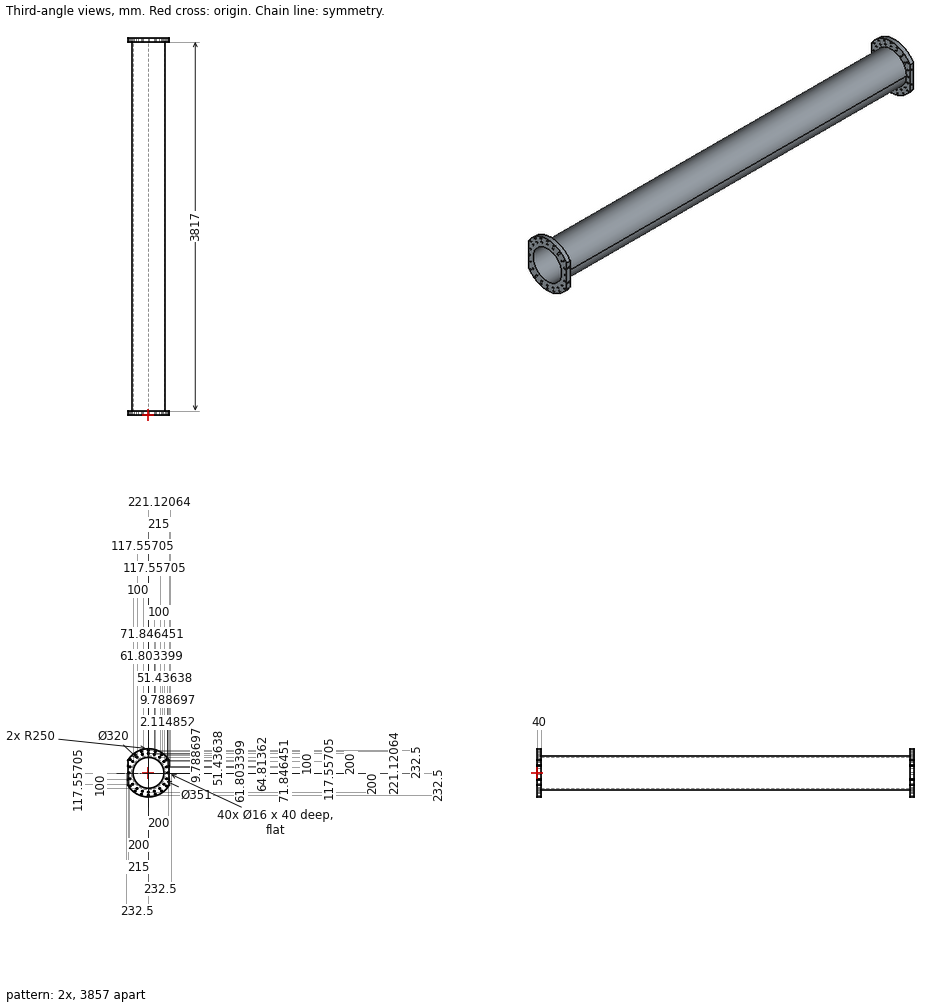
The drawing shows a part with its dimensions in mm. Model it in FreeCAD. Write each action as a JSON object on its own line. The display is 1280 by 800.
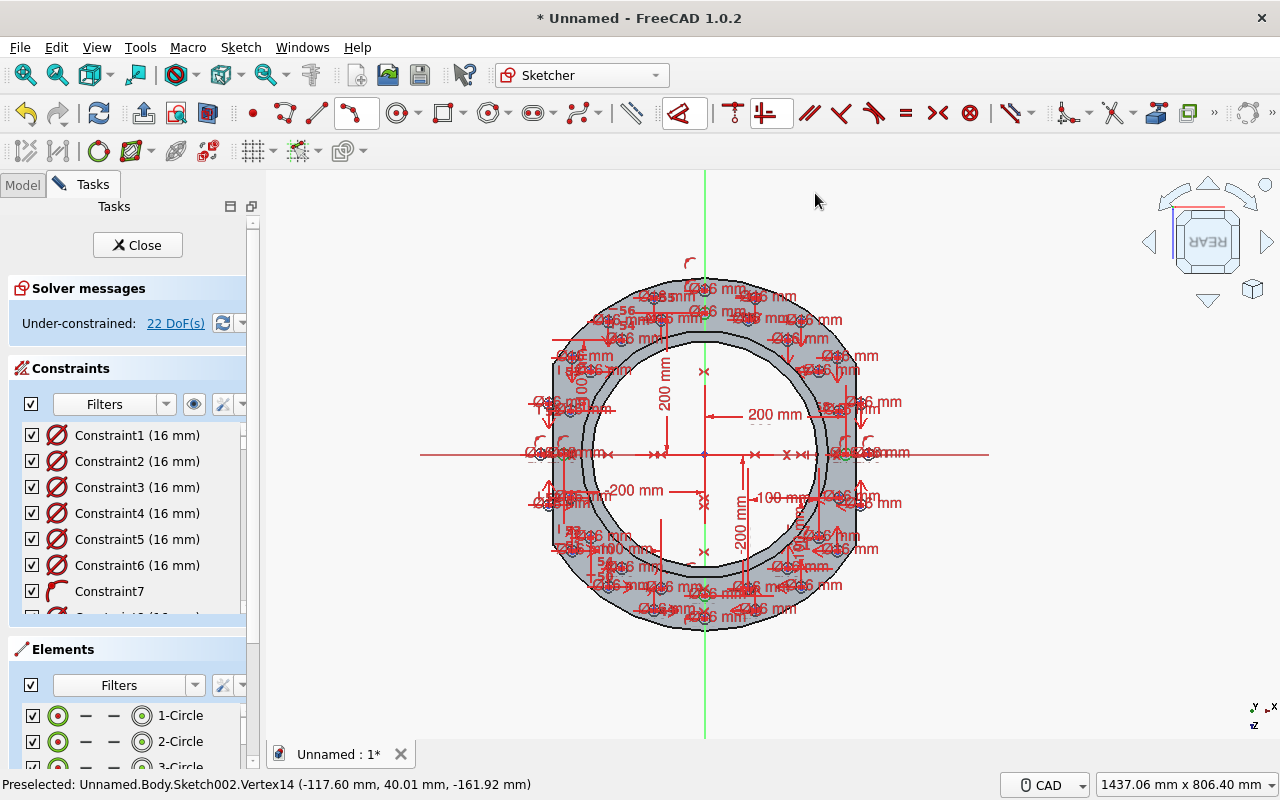
{"action": "scroll", "coordinate": [748, 320], "scroll_direction": "up", "scroll_amount": 4}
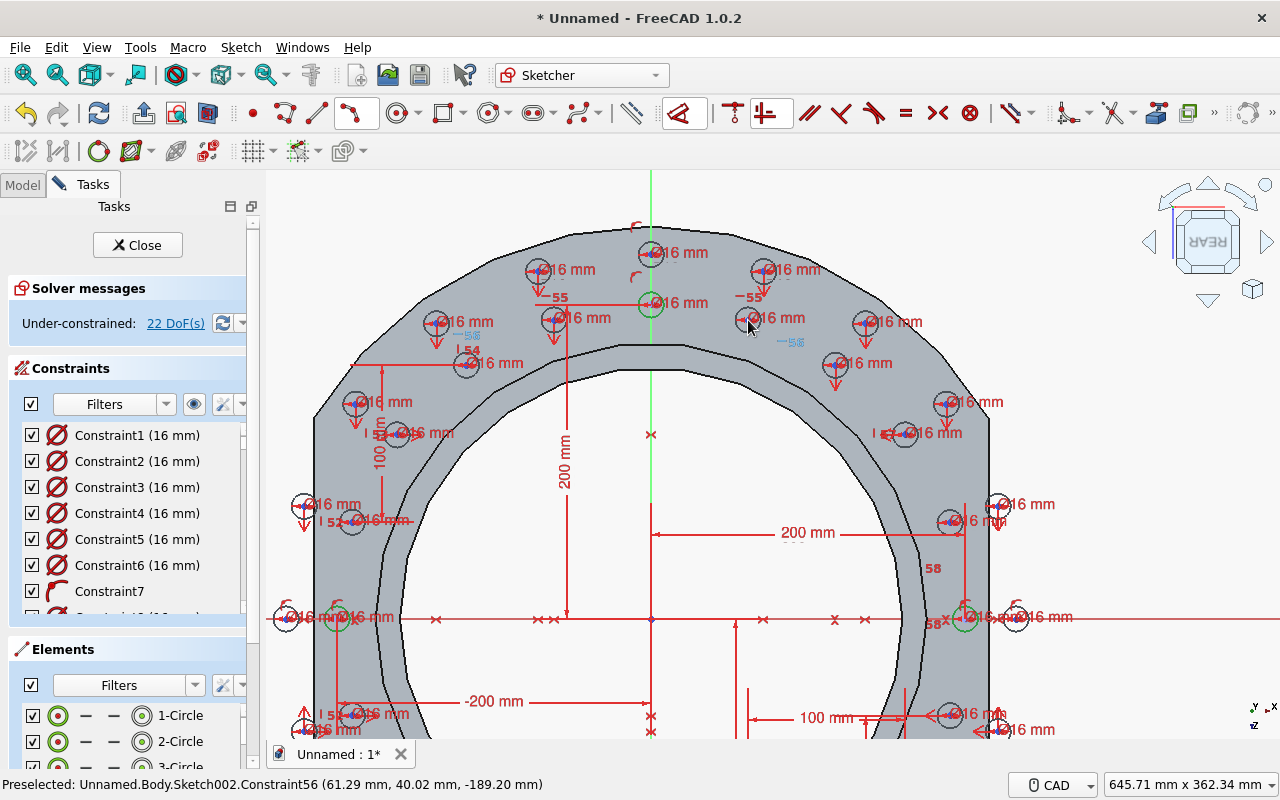
{"action": "left_click", "coordinate": [748, 320]}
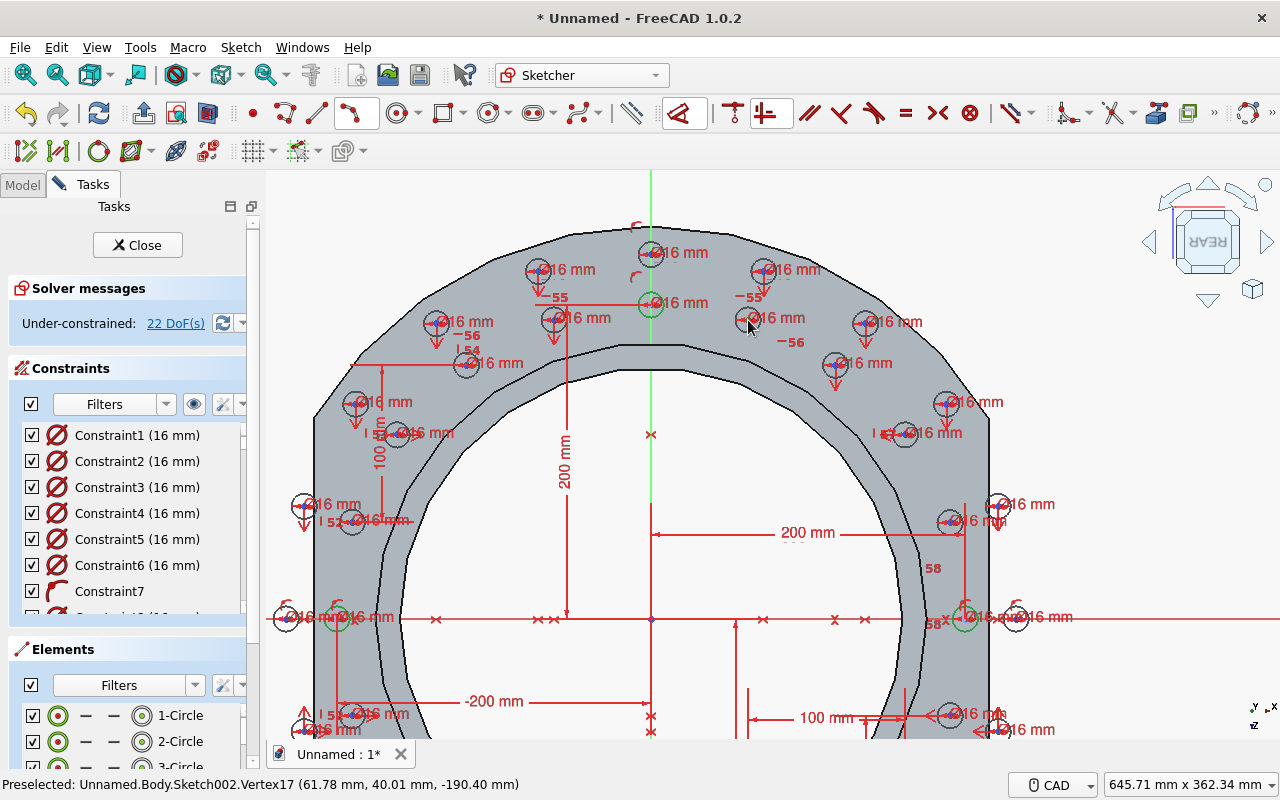
{"action": "left_click", "coordinate": [905, 435]}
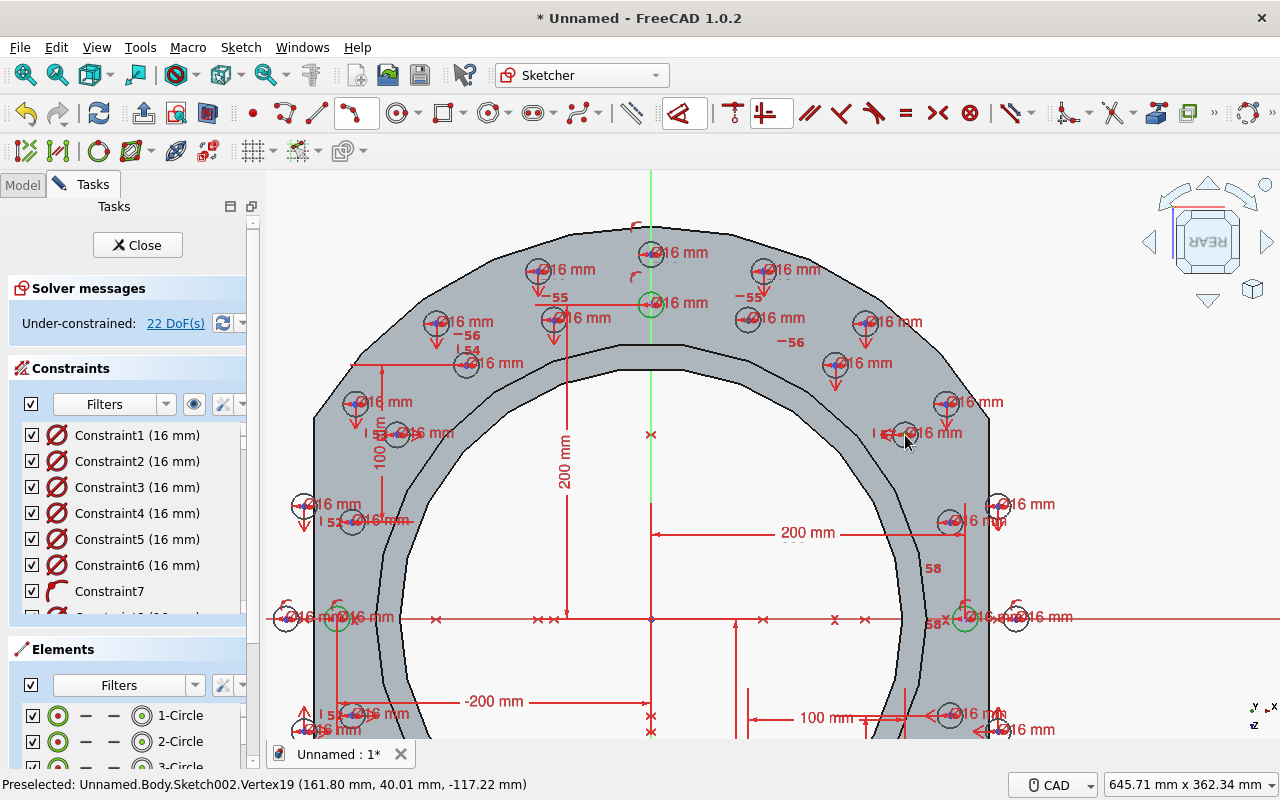
{"action": "key", "text": "l"}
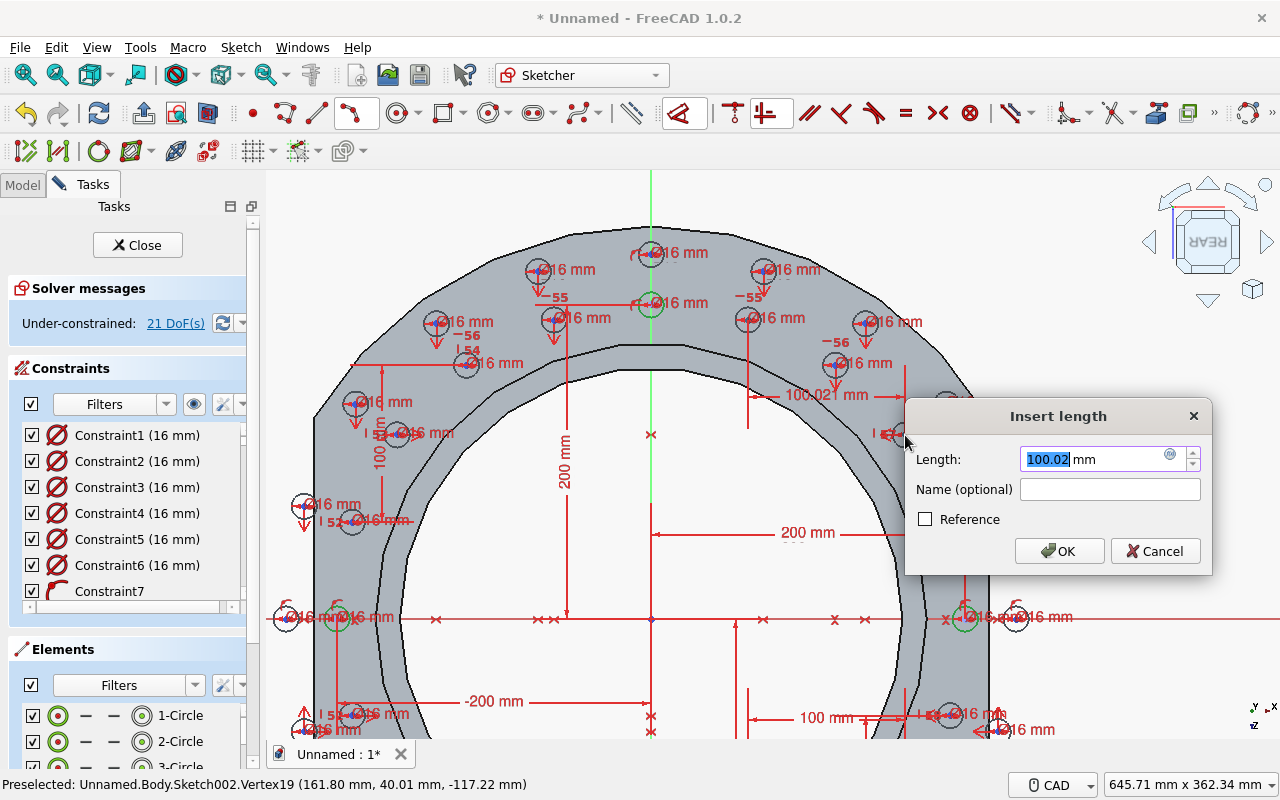
{"action": "type", "text": "100"}
{"action": "key", "text": "Return"}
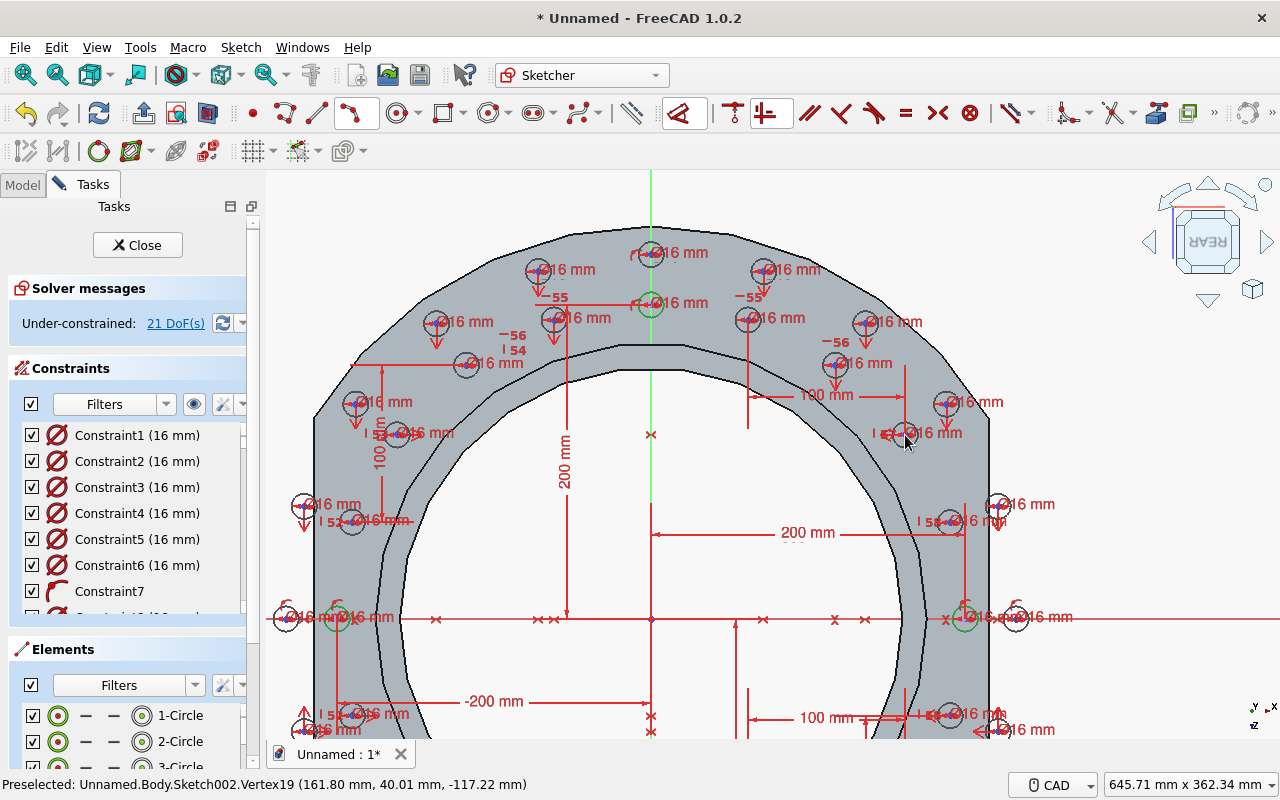
{"action": "left_click", "coordinate": [836, 365]}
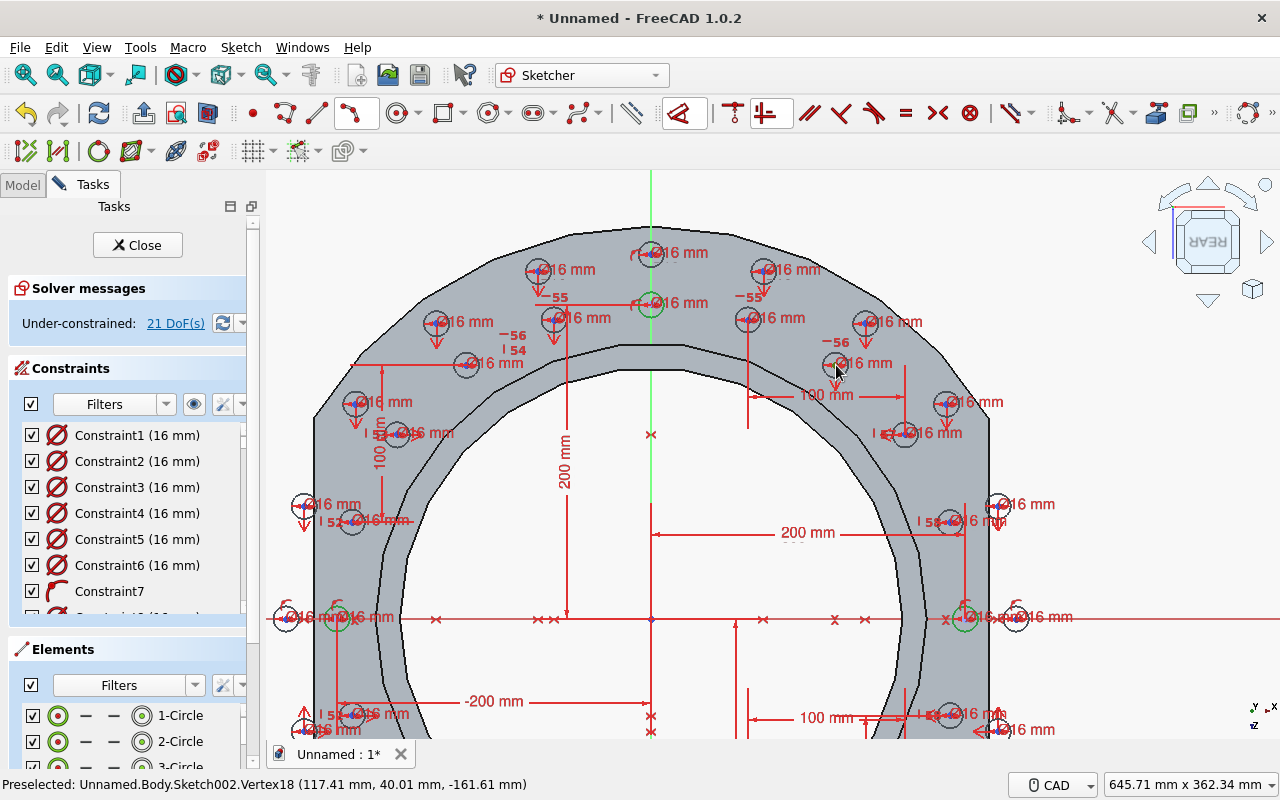
{"action": "left_click", "coordinate": [950, 523]}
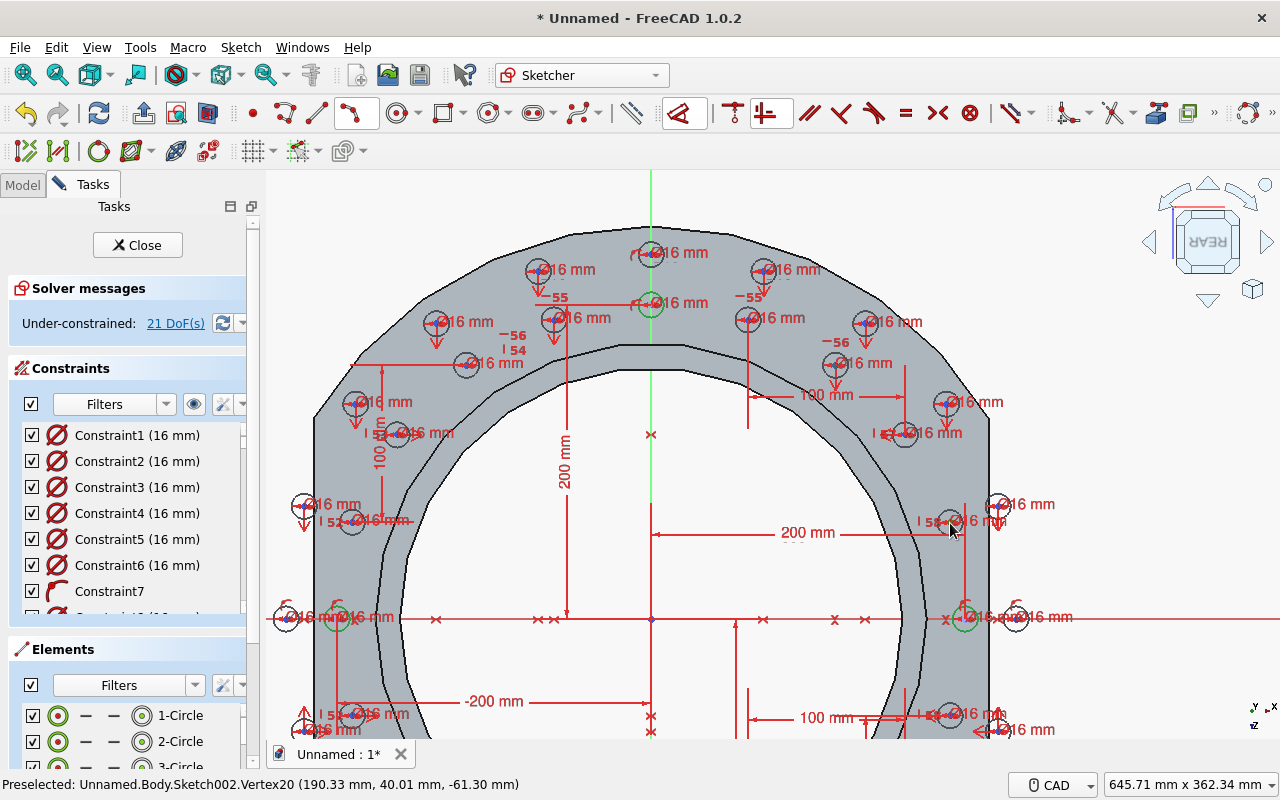
{"action": "key", "text": "i"}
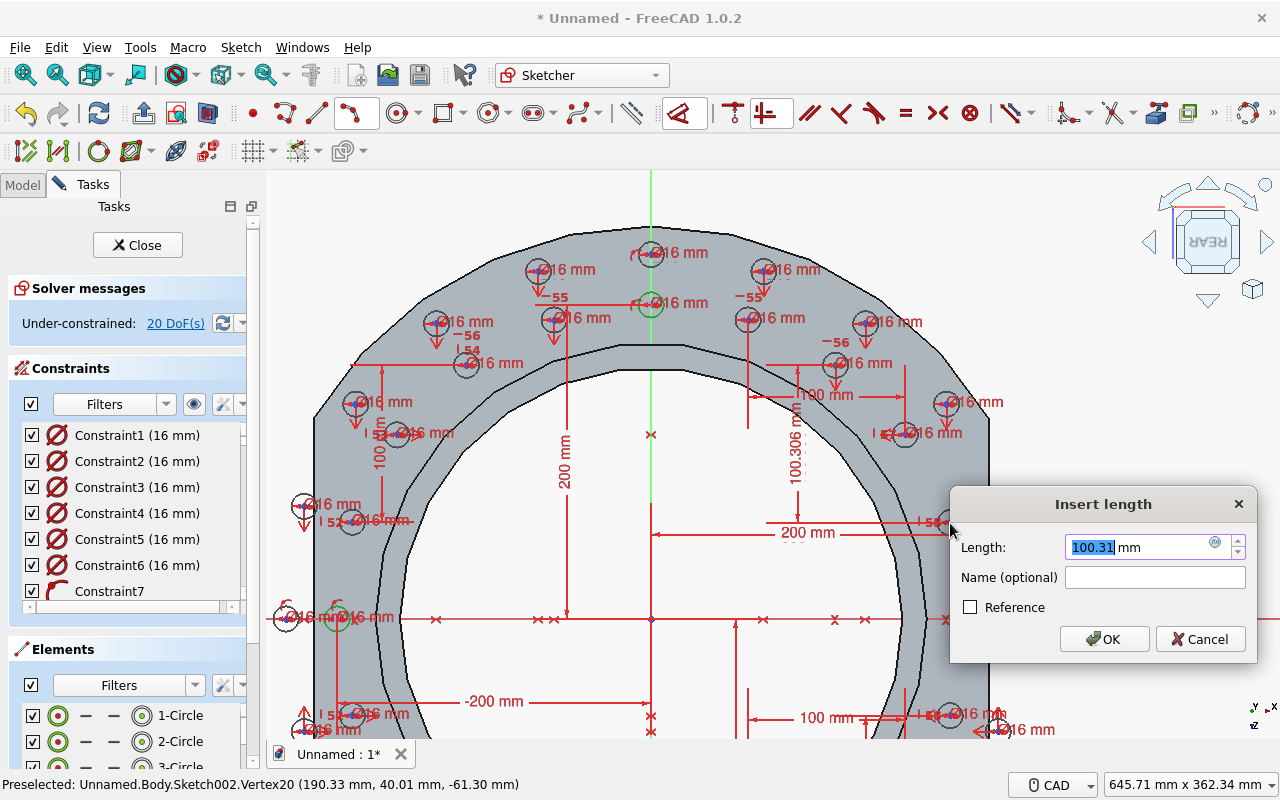
{"action": "type", "text": "100"}
{"action": "key", "text": "Return"}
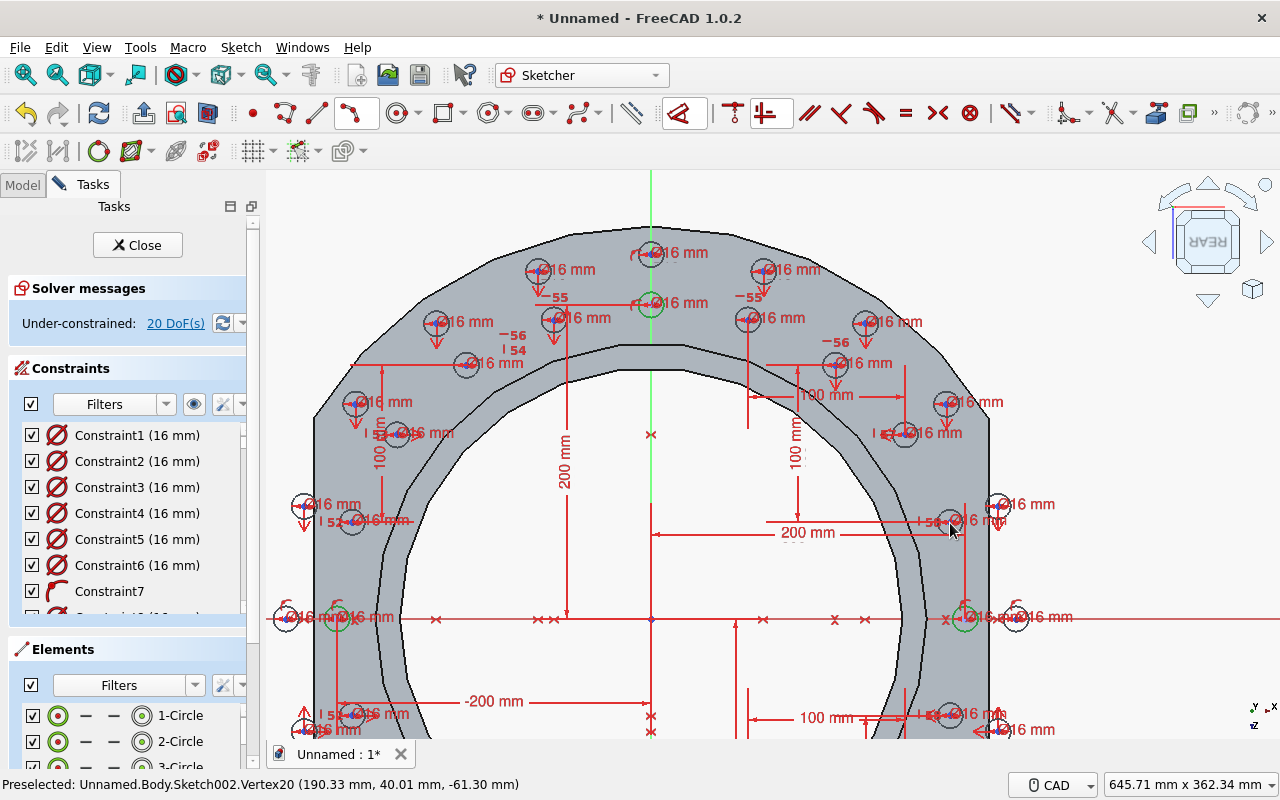
{"action": "left_click", "coordinate": [1016, 619]}